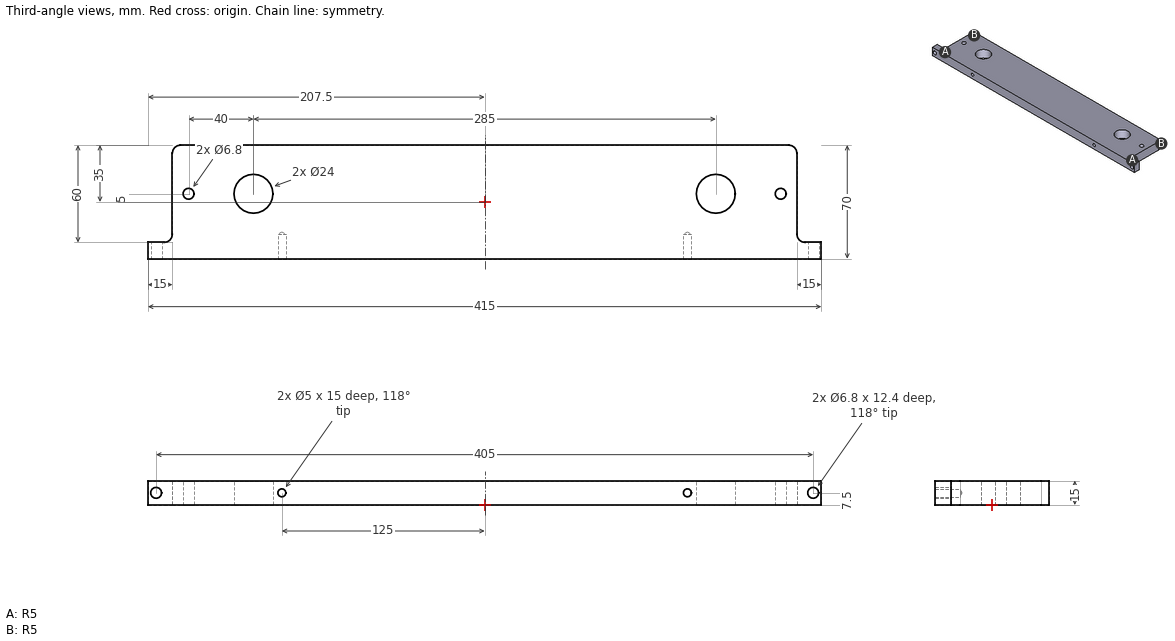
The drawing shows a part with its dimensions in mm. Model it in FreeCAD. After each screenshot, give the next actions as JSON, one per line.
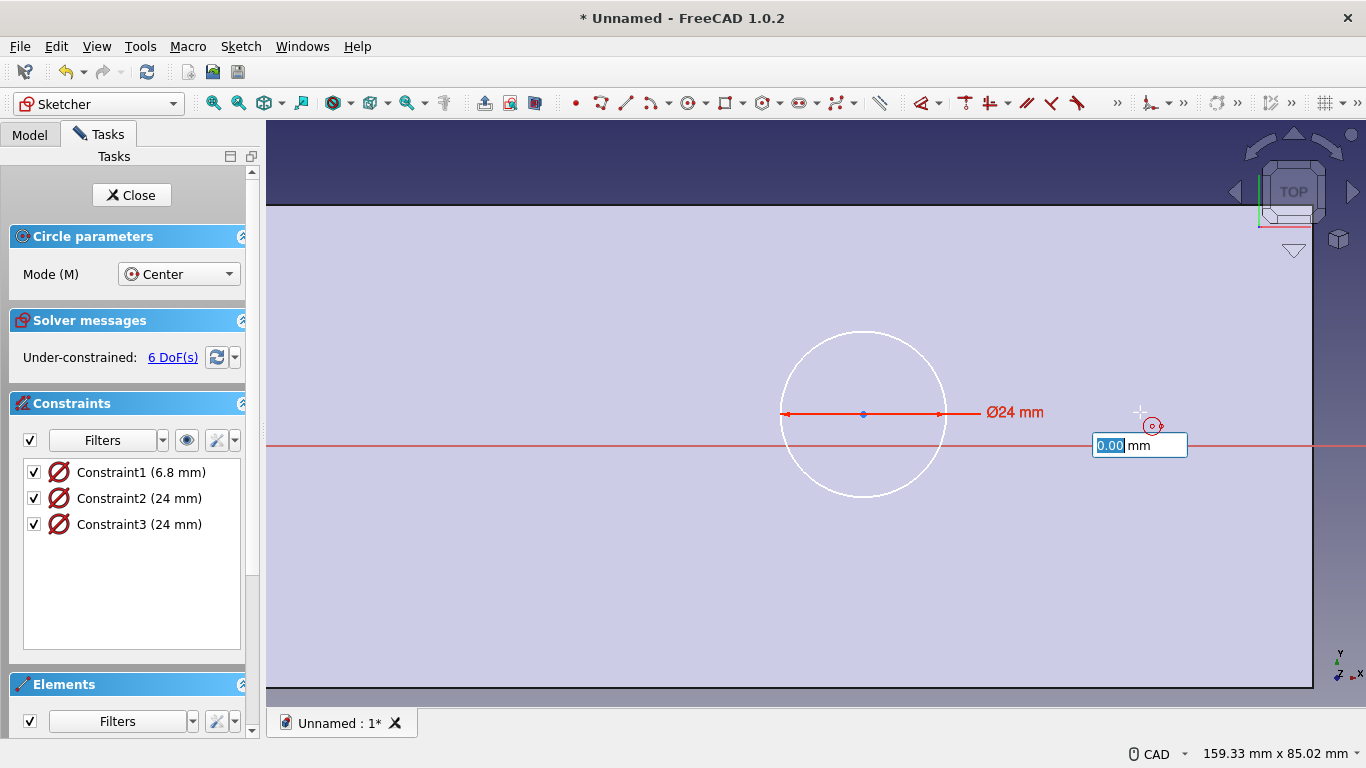
{"action": "scroll", "coordinate": [1031, 414], "scroll_direction": "down", "scroll_amount": 7}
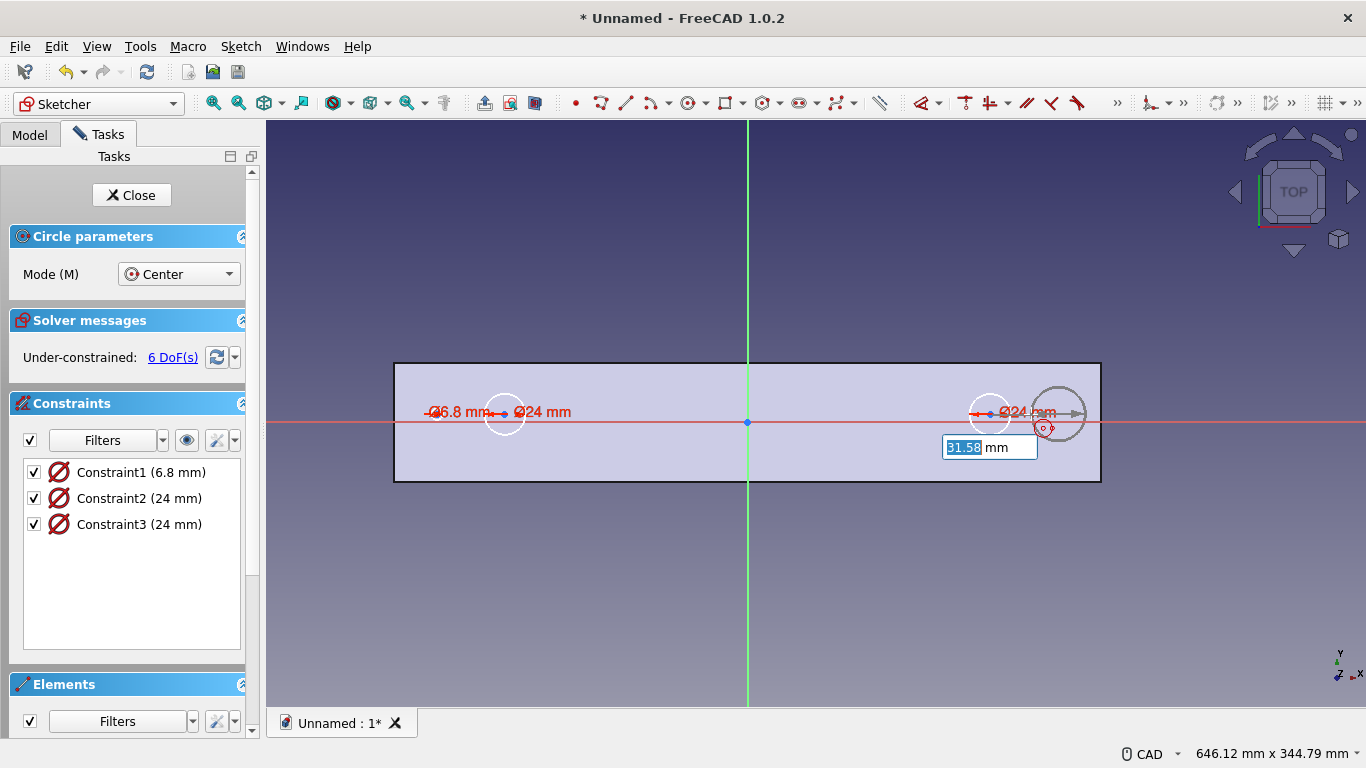
{"action": "scroll", "coordinate": [1063, 410], "scroll_direction": "up", "scroll_amount": 2}
{"action": "mouse_move", "coordinate": [1062, 409]}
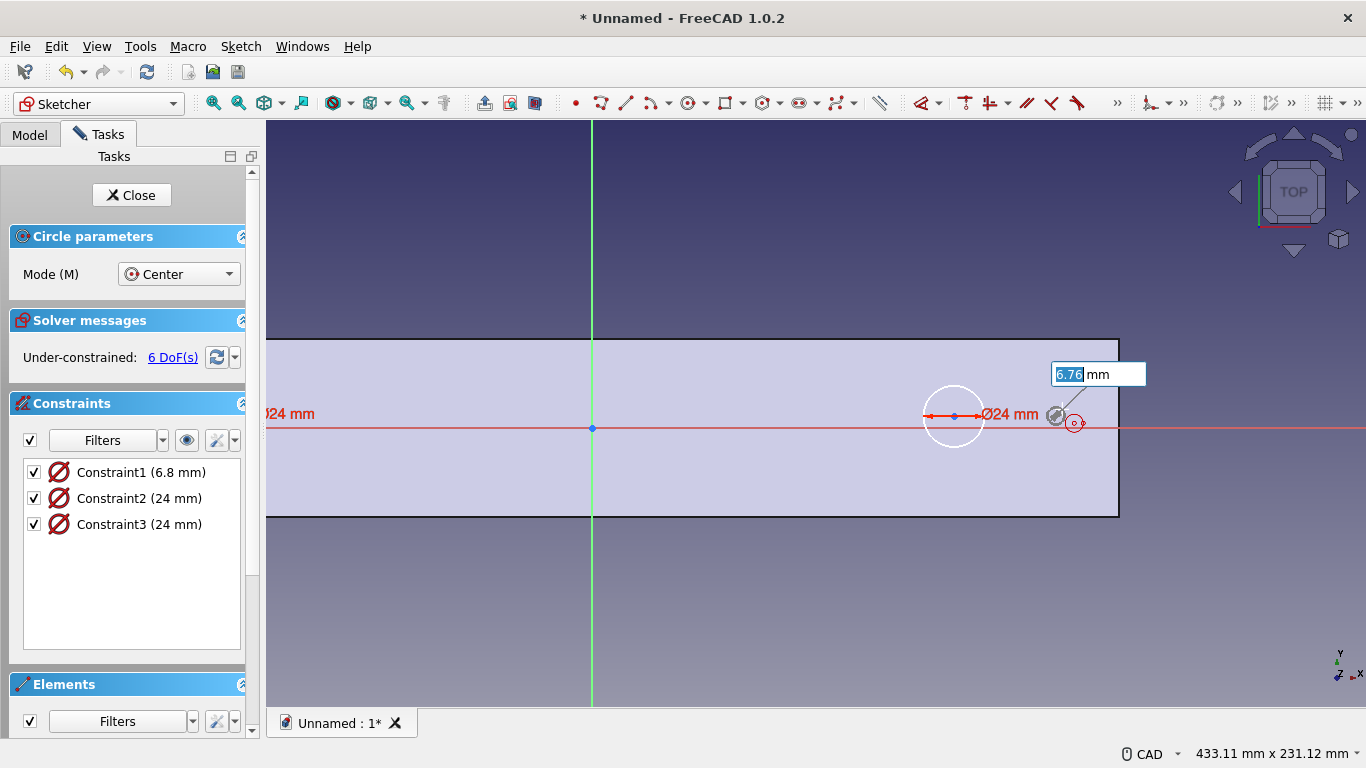
{"action": "type", "text": "6.8"}
{"action": "key", "text": "Return"}
{"action": "key", "text": "Escape"}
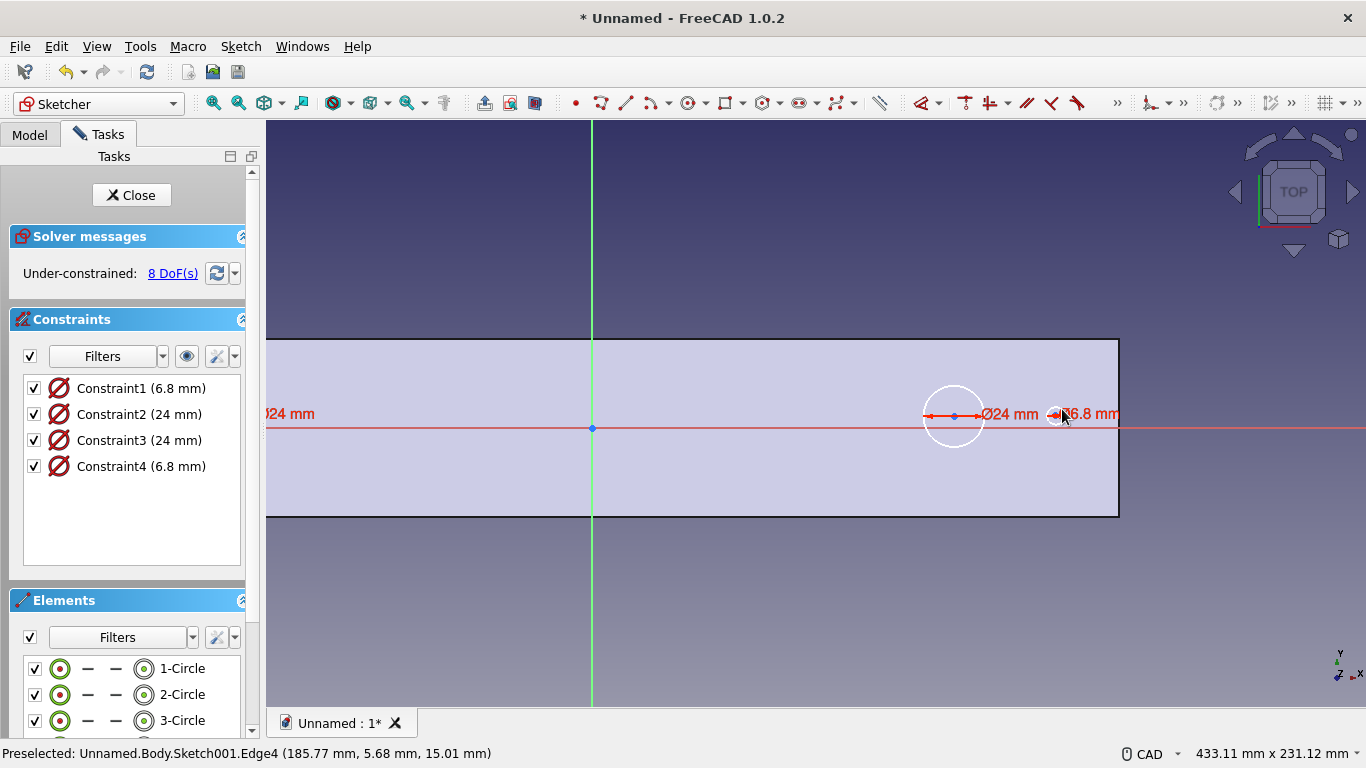
{"action": "scroll", "coordinate": [1063, 409], "scroll_direction": "down", "scroll_amount": 2}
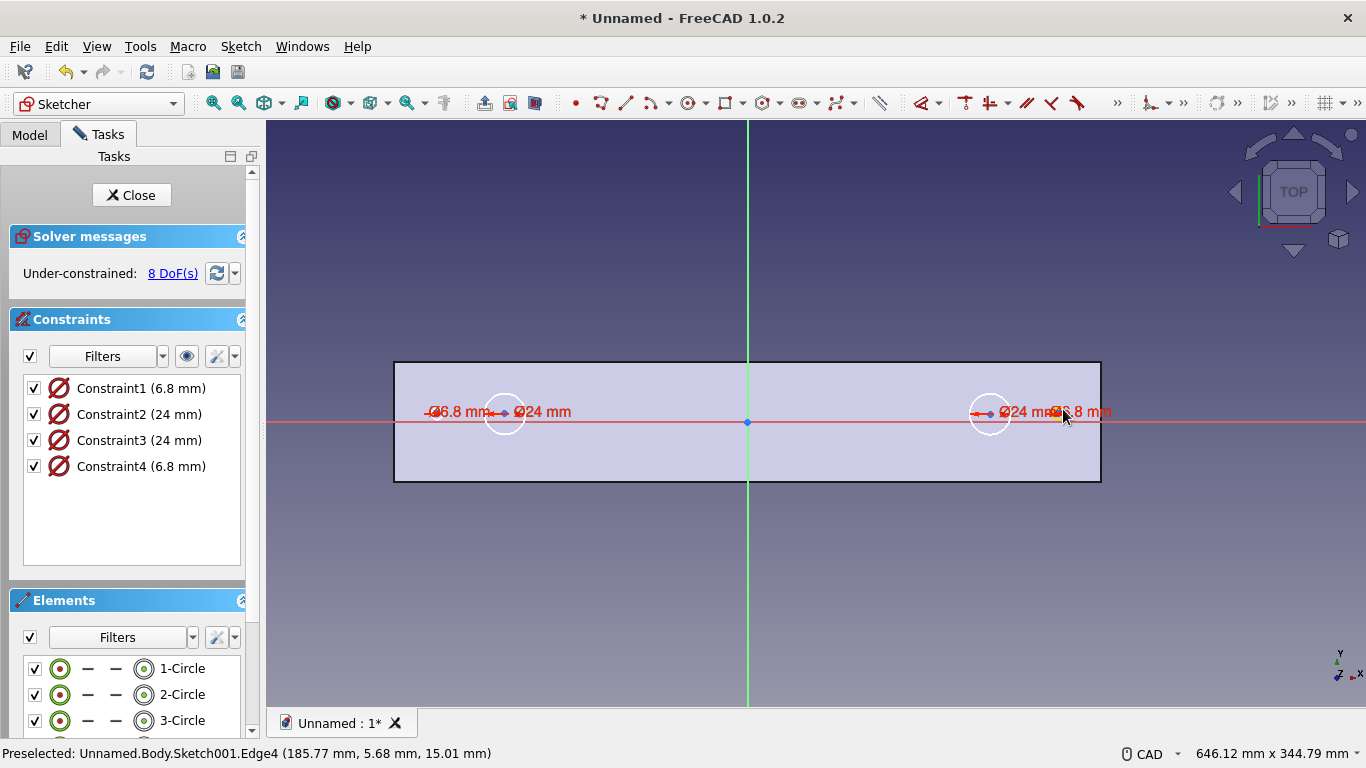
{"action": "left_click", "coordinate": [505, 414]}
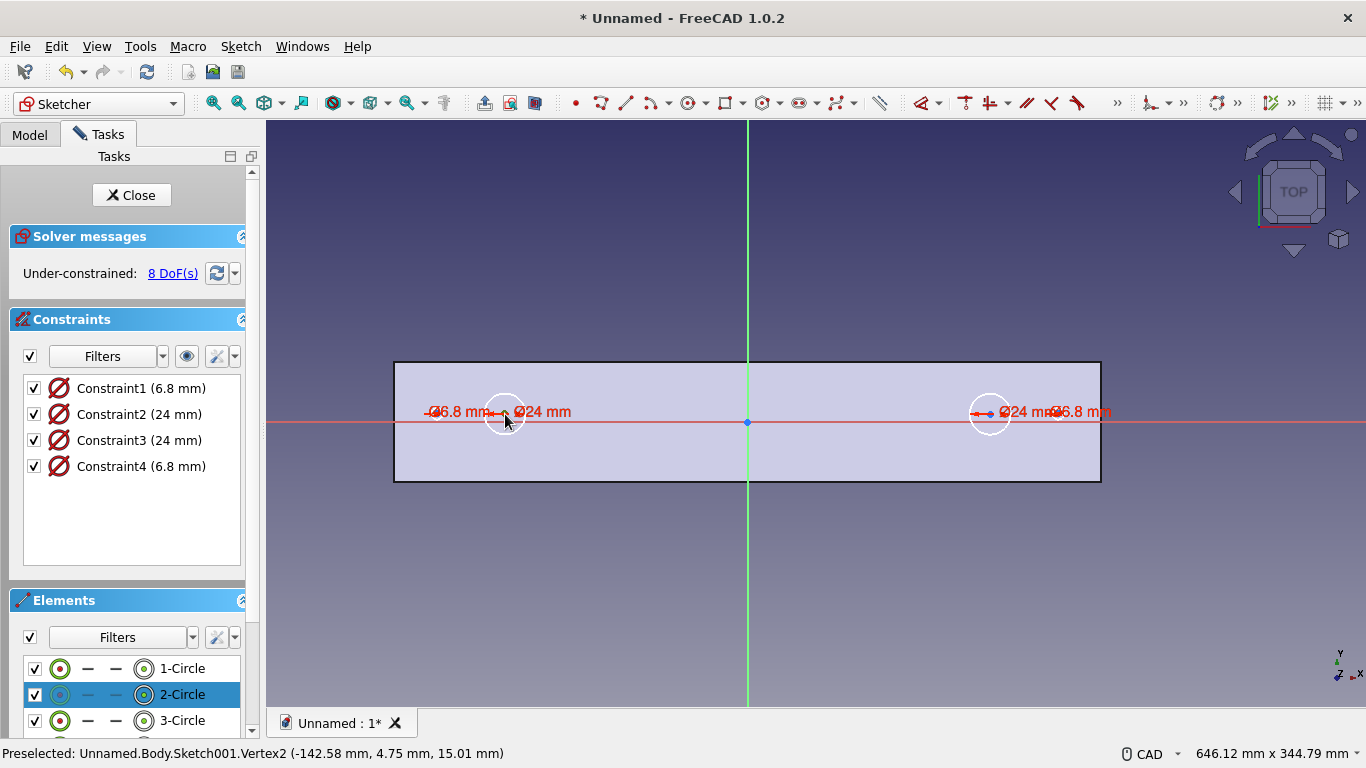
{"action": "left_click", "coordinate": [990, 414]}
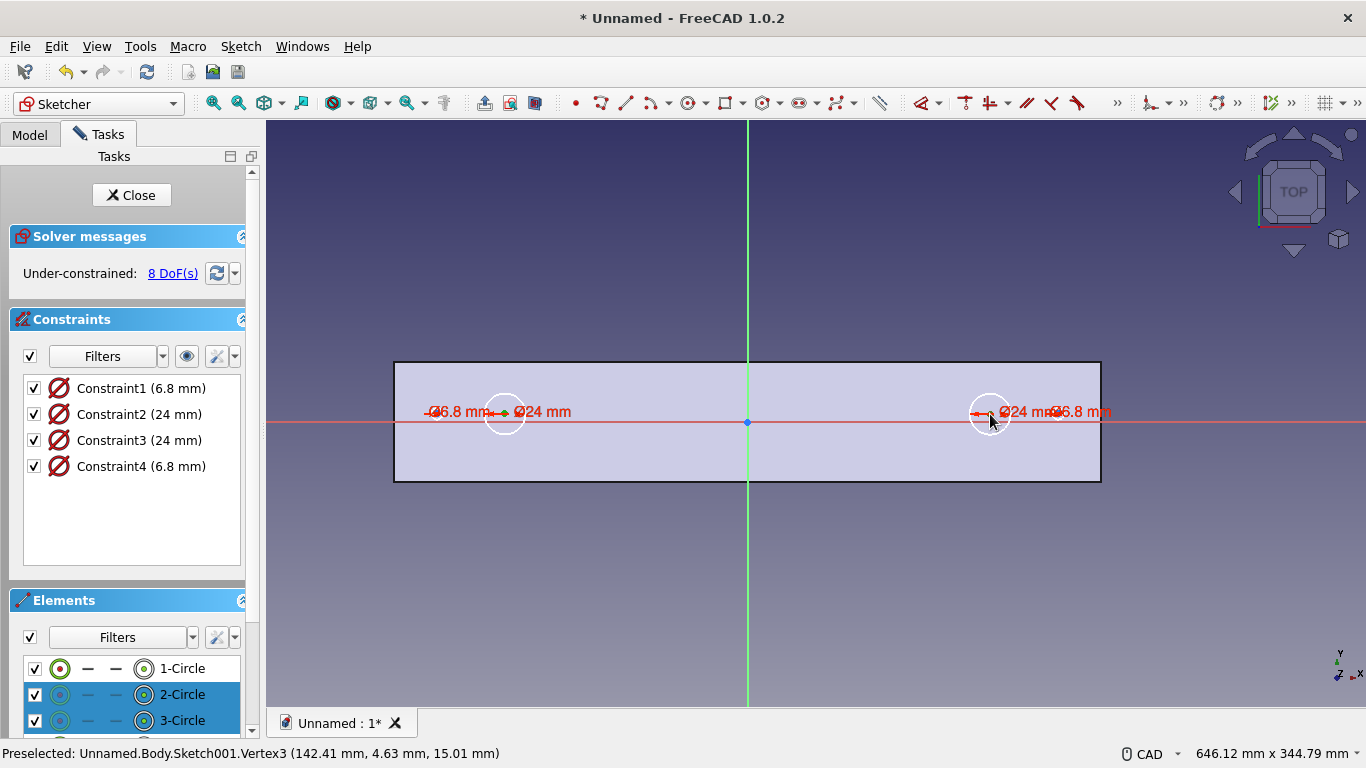
{"action": "left_click", "coordinate": [748, 641]}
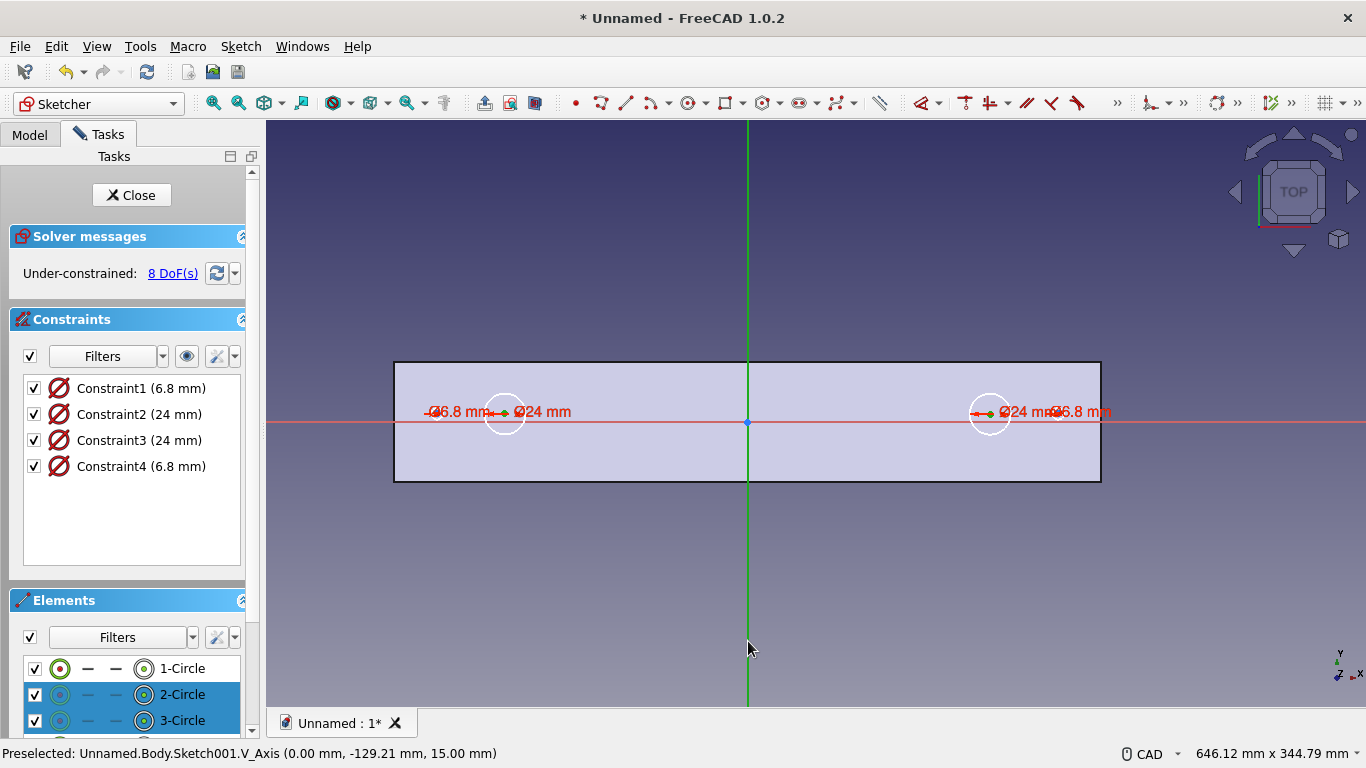
{"action": "key", "text": "s"}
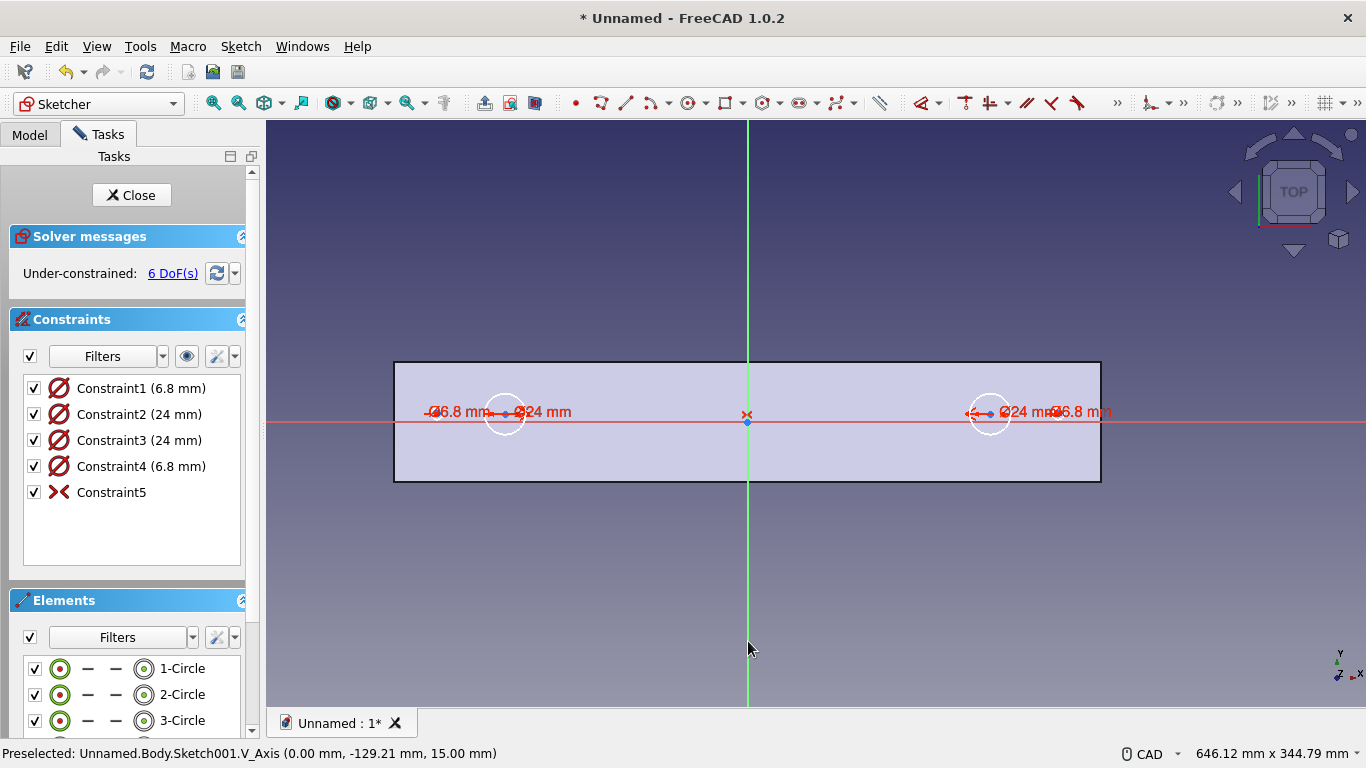
{"action": "left_click", "coordinate": [437, 414]}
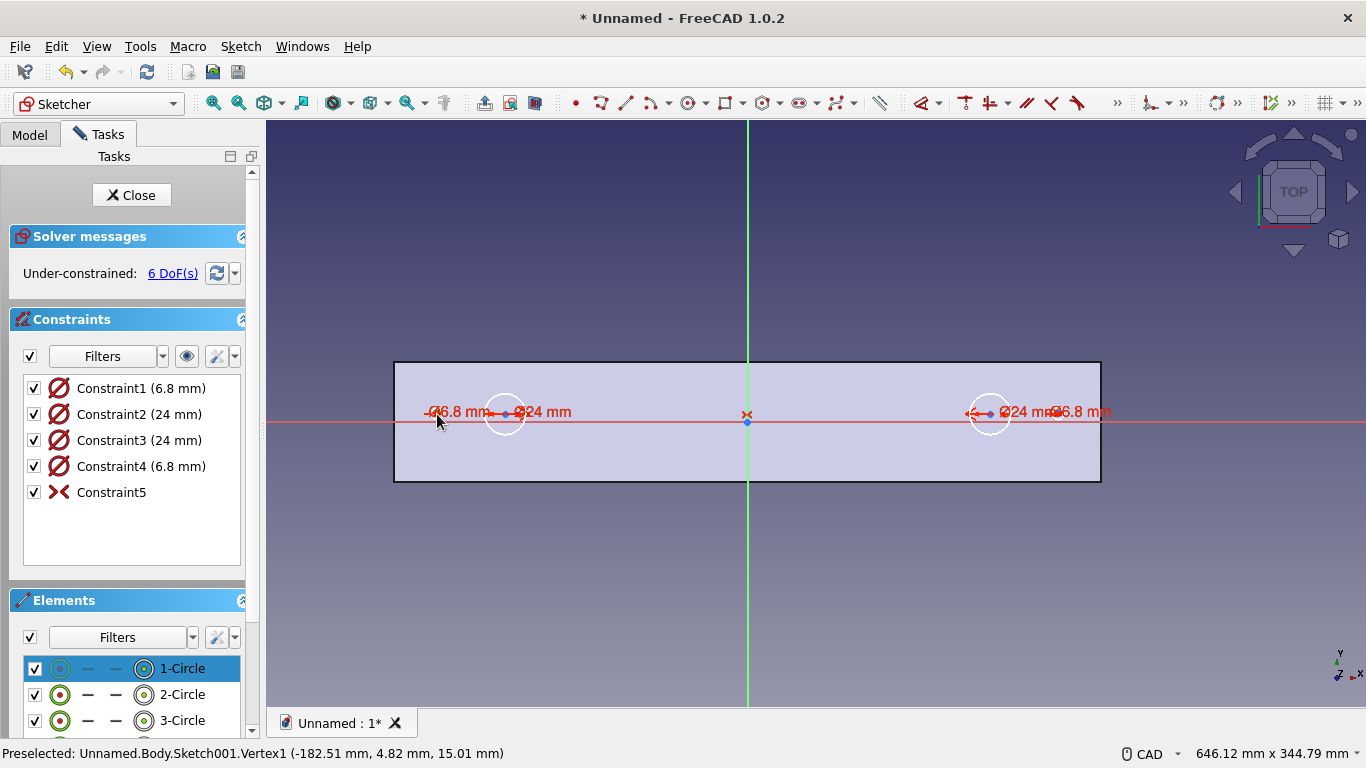
{"action": "left_click", "coordinate": [1058, 414]}